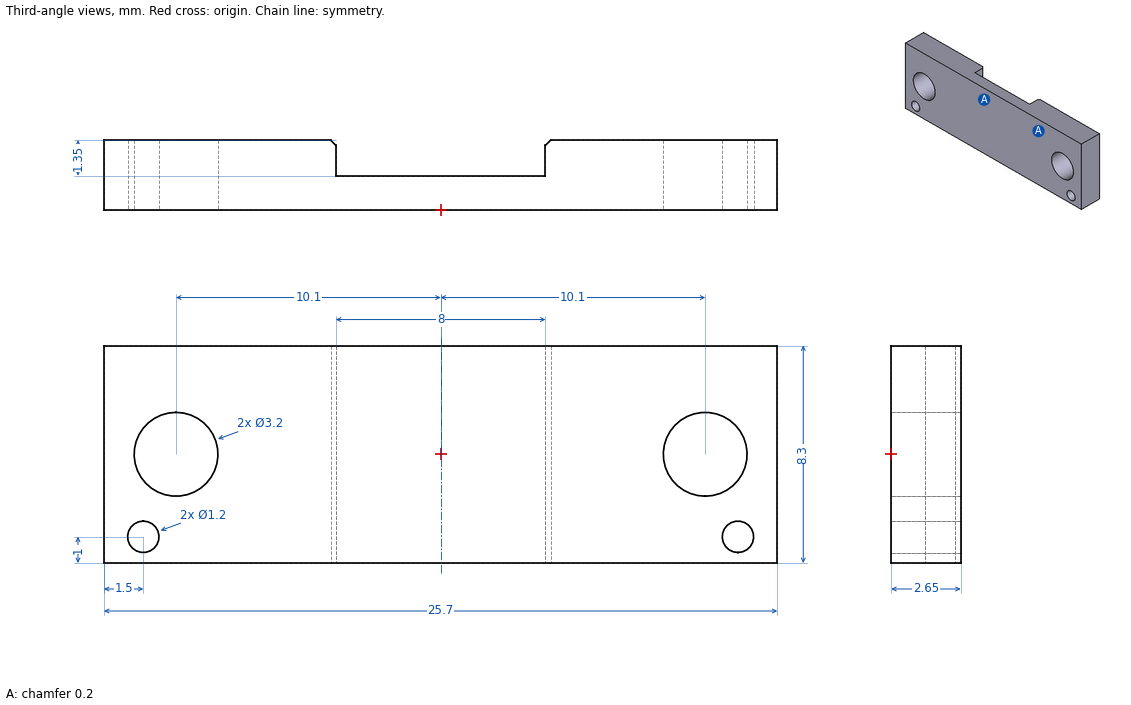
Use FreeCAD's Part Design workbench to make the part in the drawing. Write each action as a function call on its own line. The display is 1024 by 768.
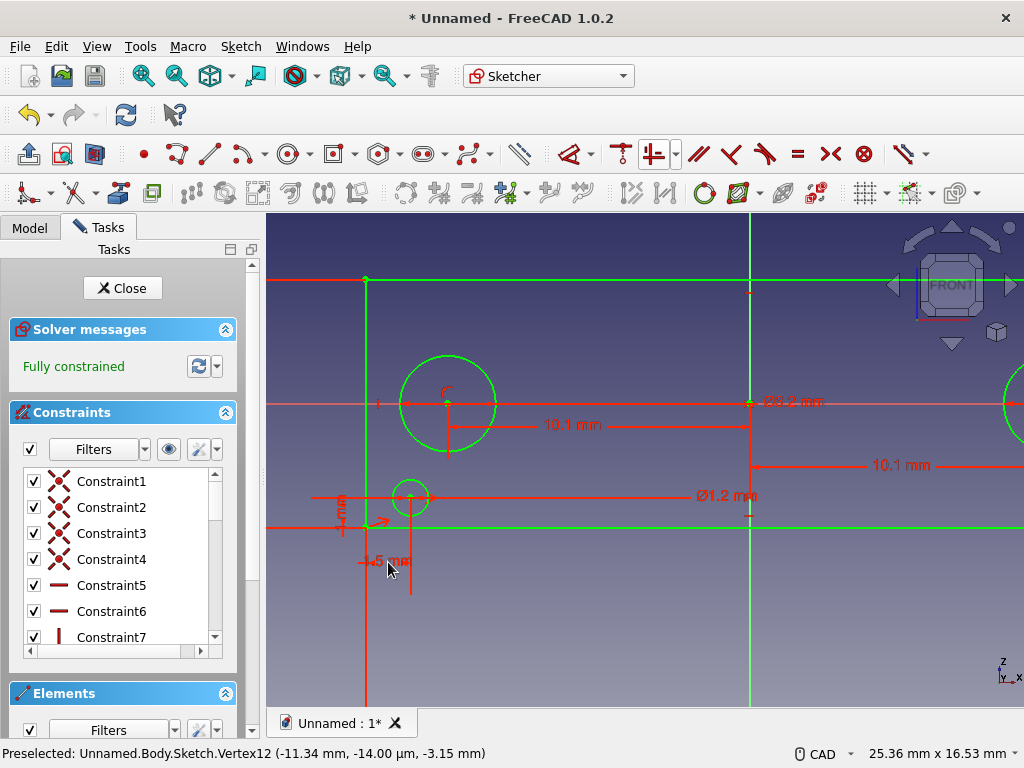
click(123, 288)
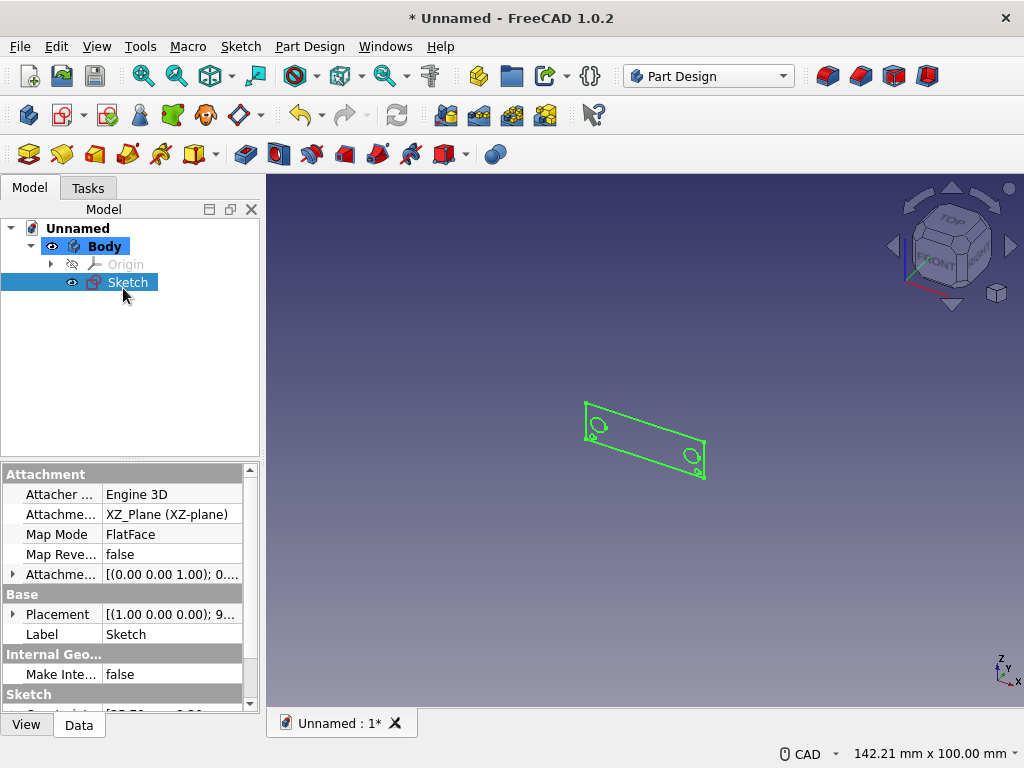
click(29, 154)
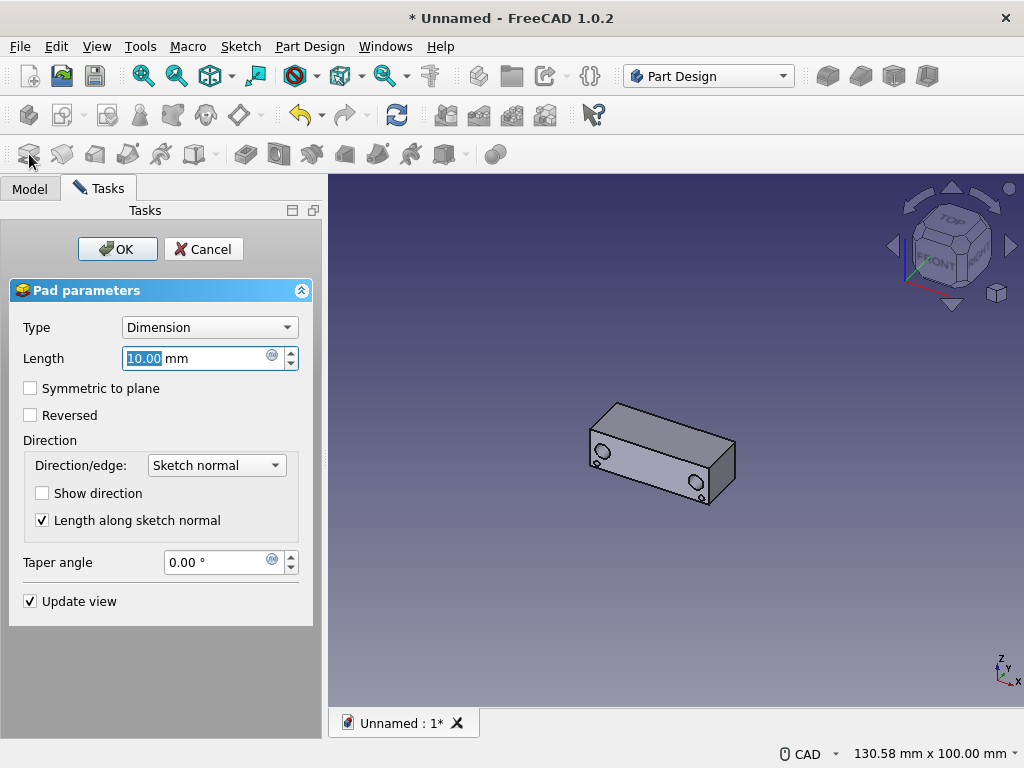
text(2.65)
key(Tab)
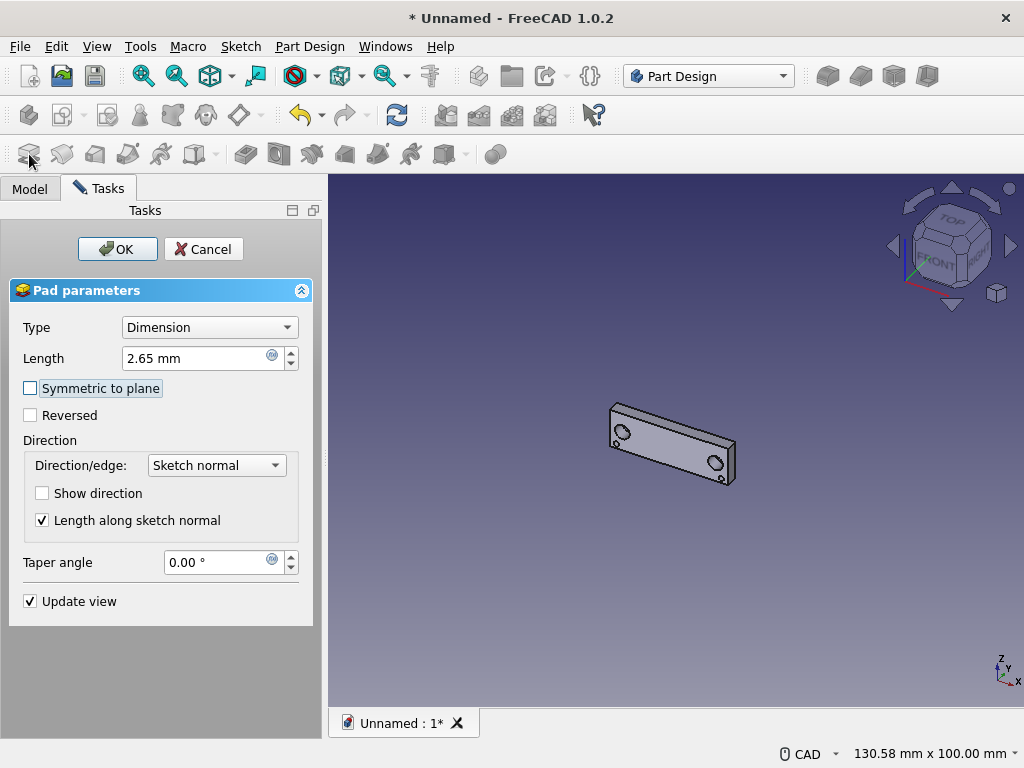
click(31, 415)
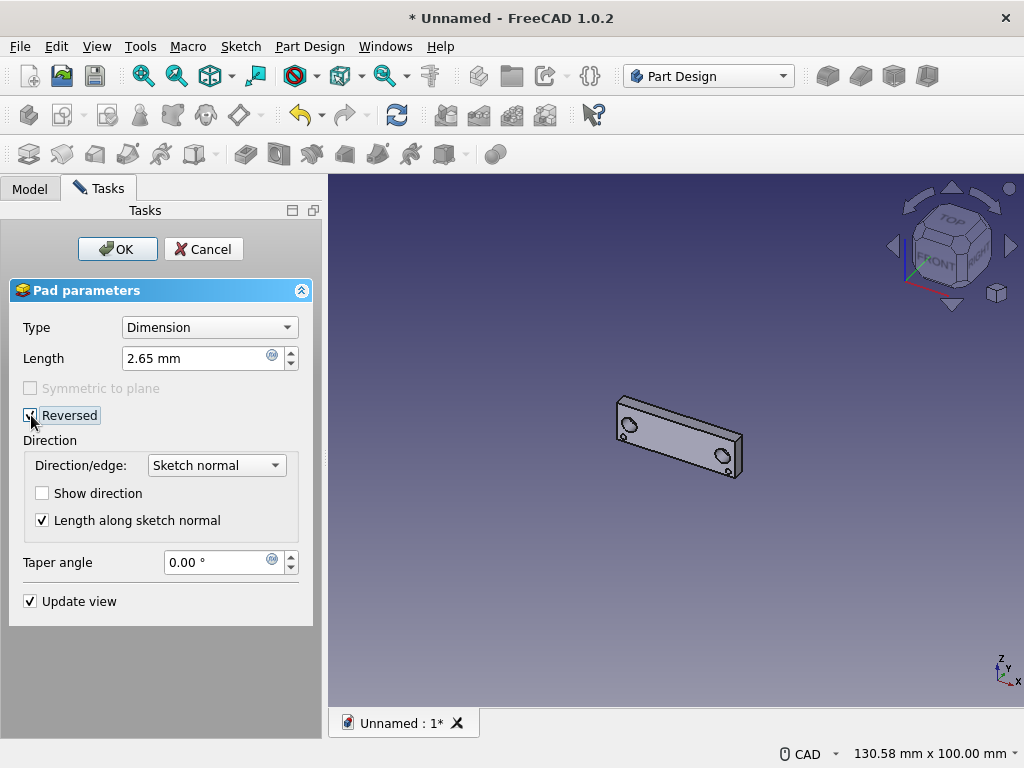
click(118, 249)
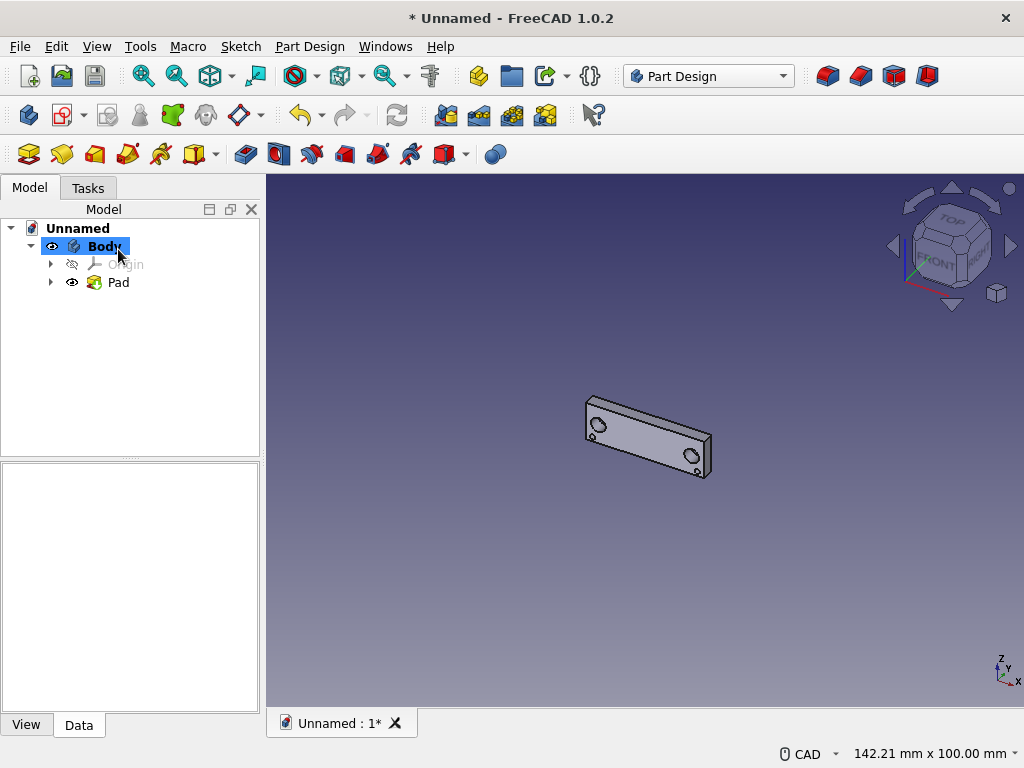
click(144, 76)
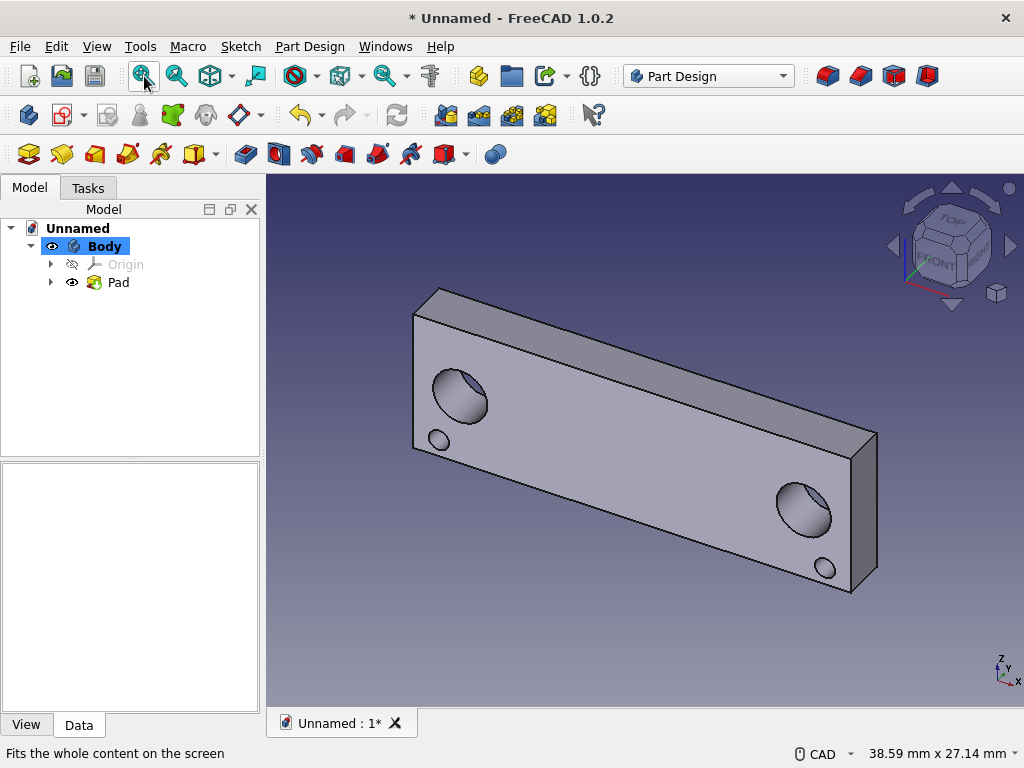
key(4)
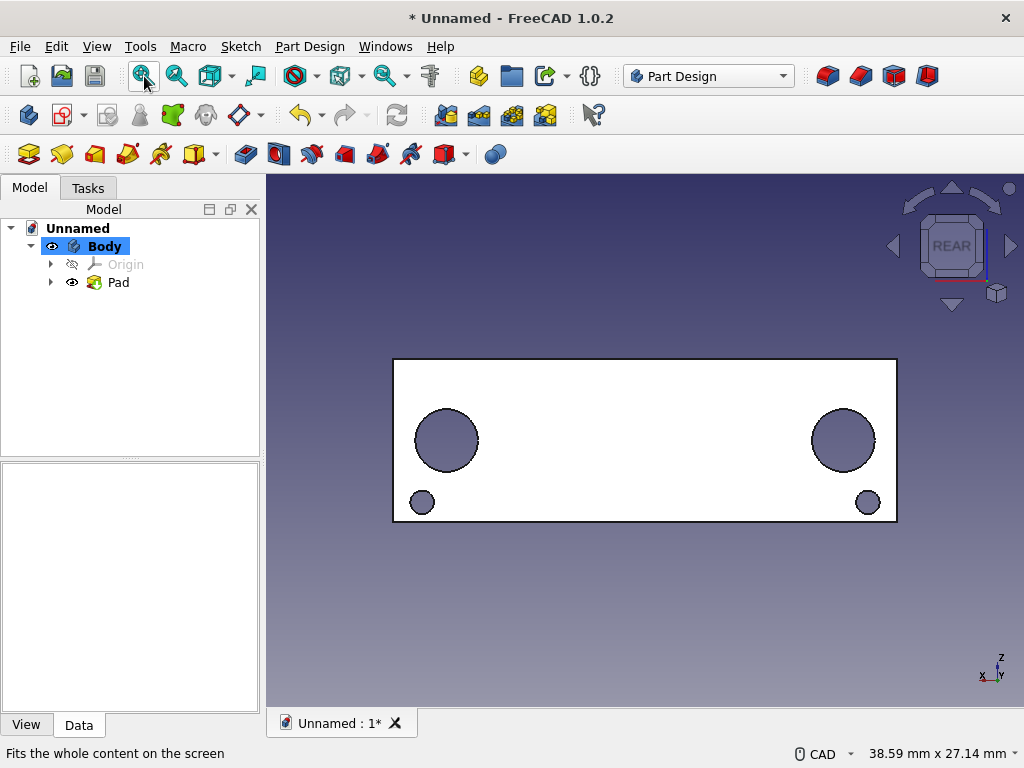
click(573, 439)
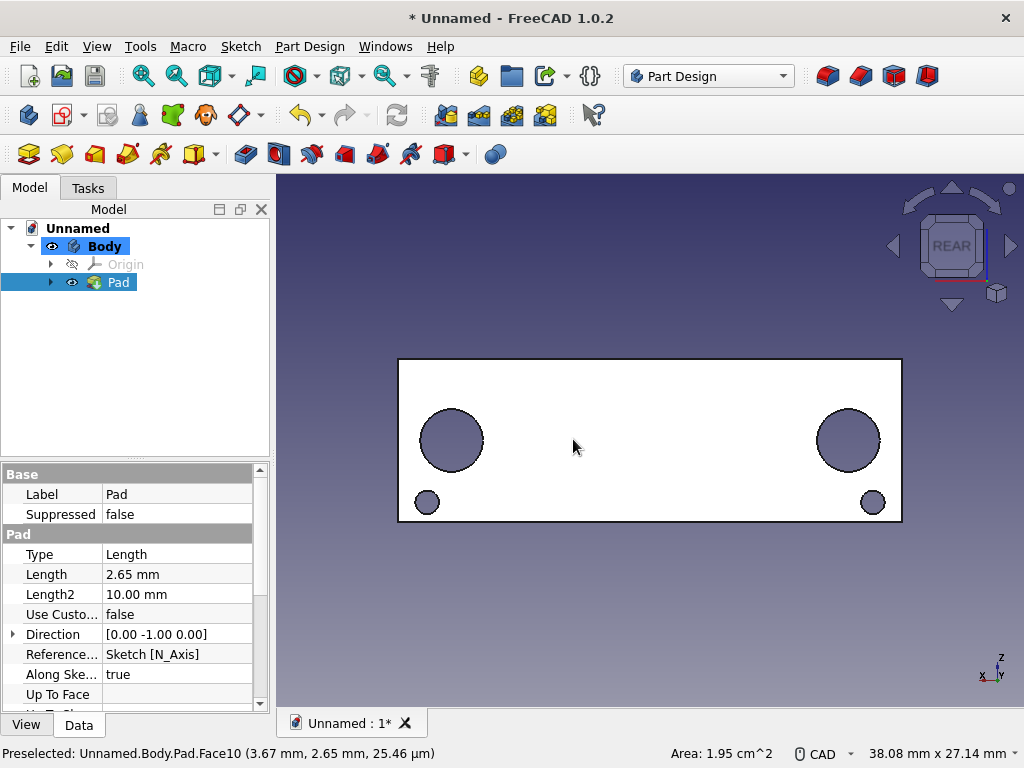
click(62, 116)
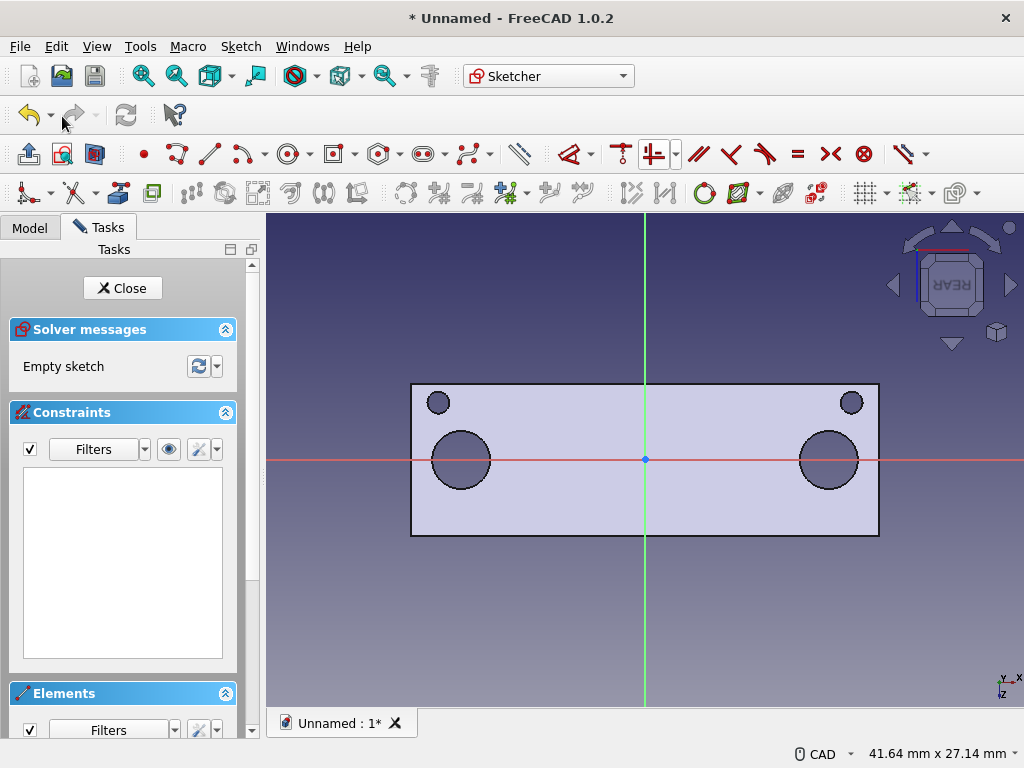
scroll(701, 460, up, 4)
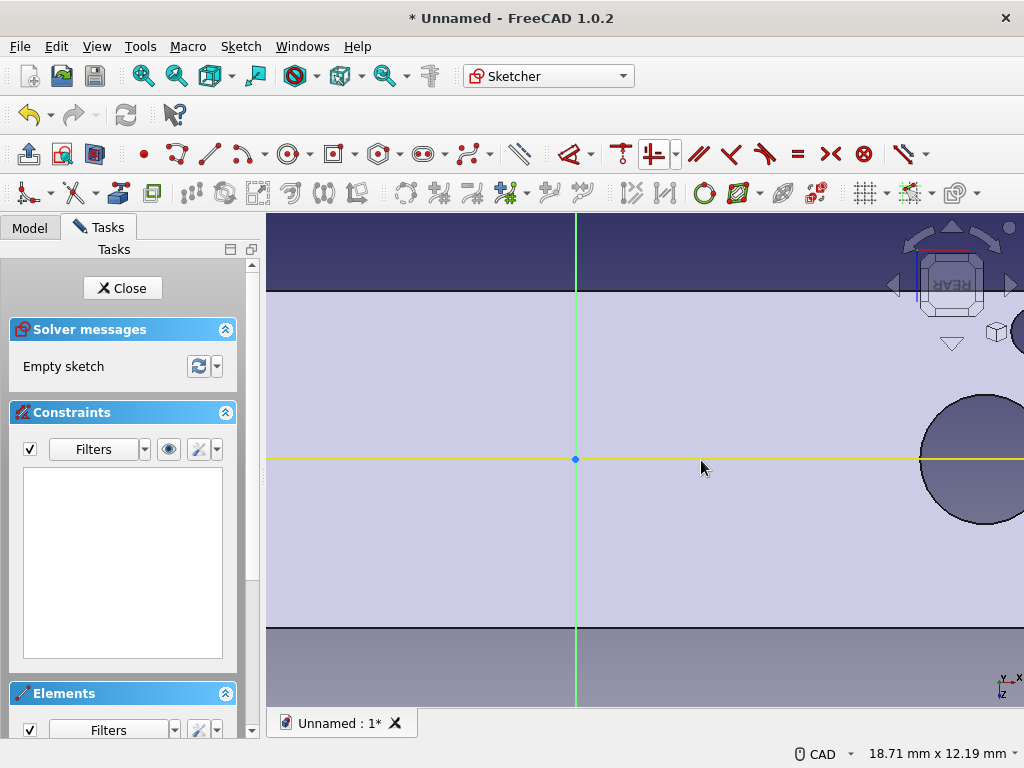
click(332, 154)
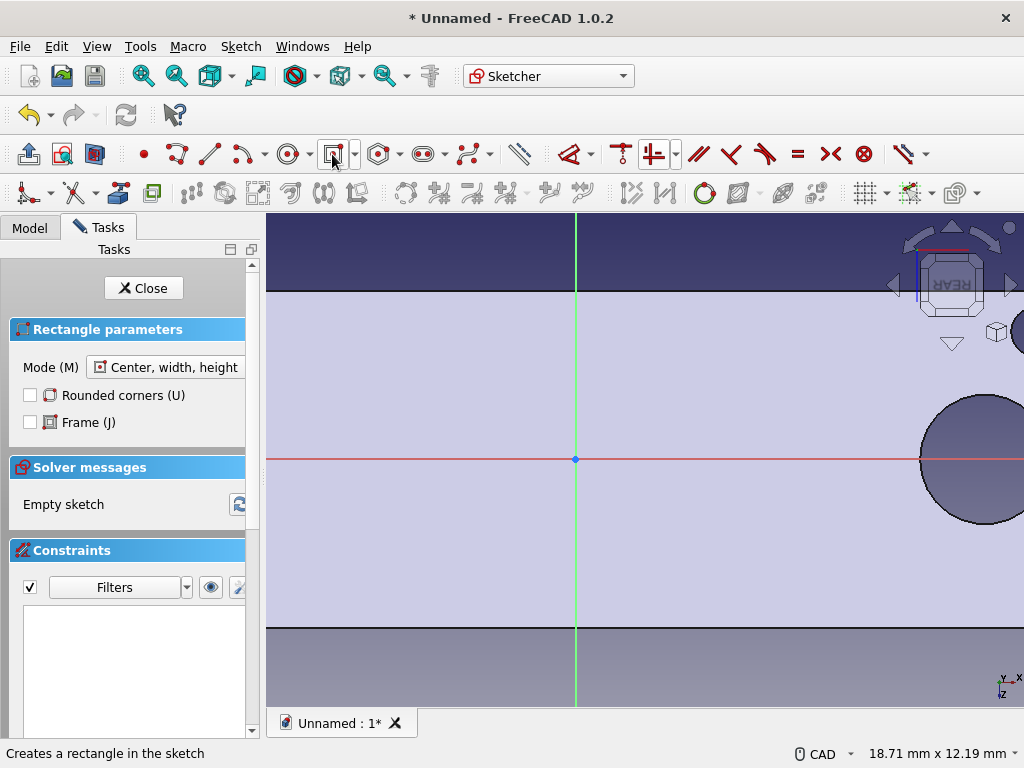
click(576, 459)
move(738, 291)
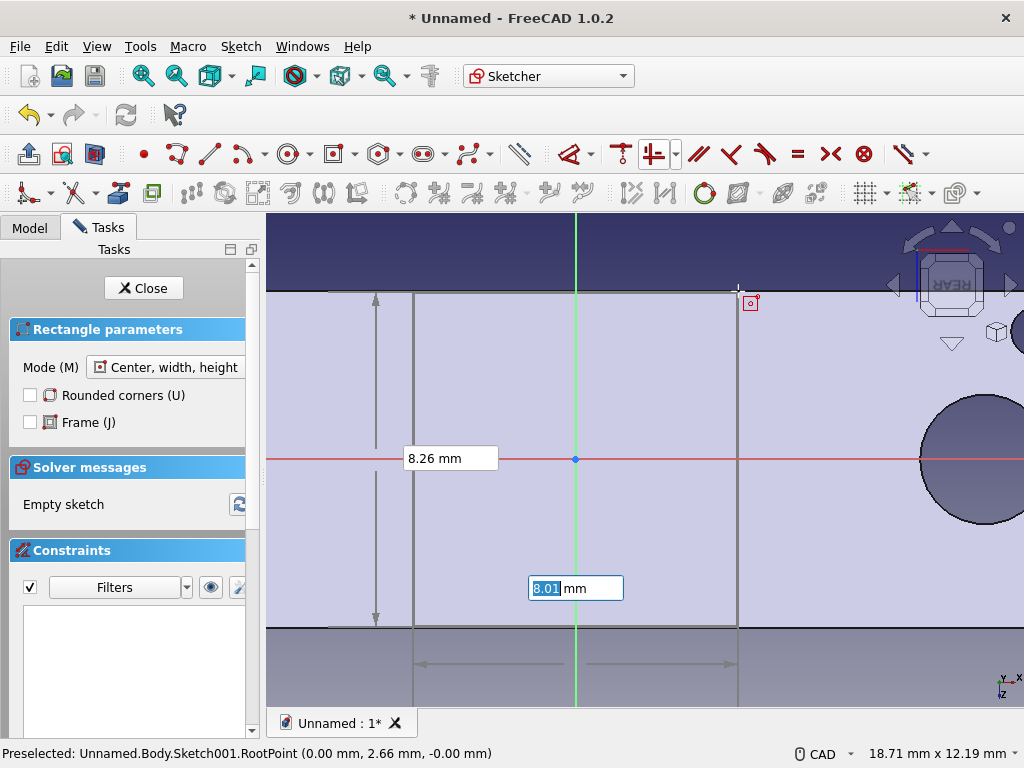
text(8)
key(Tab)
text(8.3)
key(Return)
key(Escape)